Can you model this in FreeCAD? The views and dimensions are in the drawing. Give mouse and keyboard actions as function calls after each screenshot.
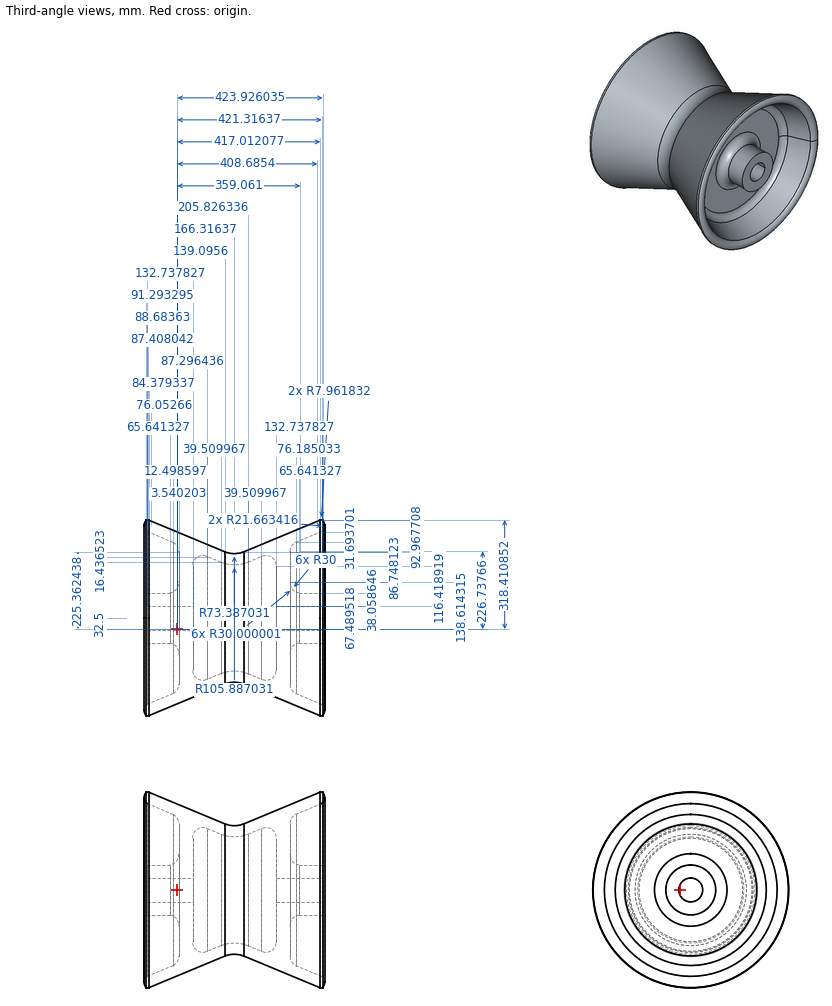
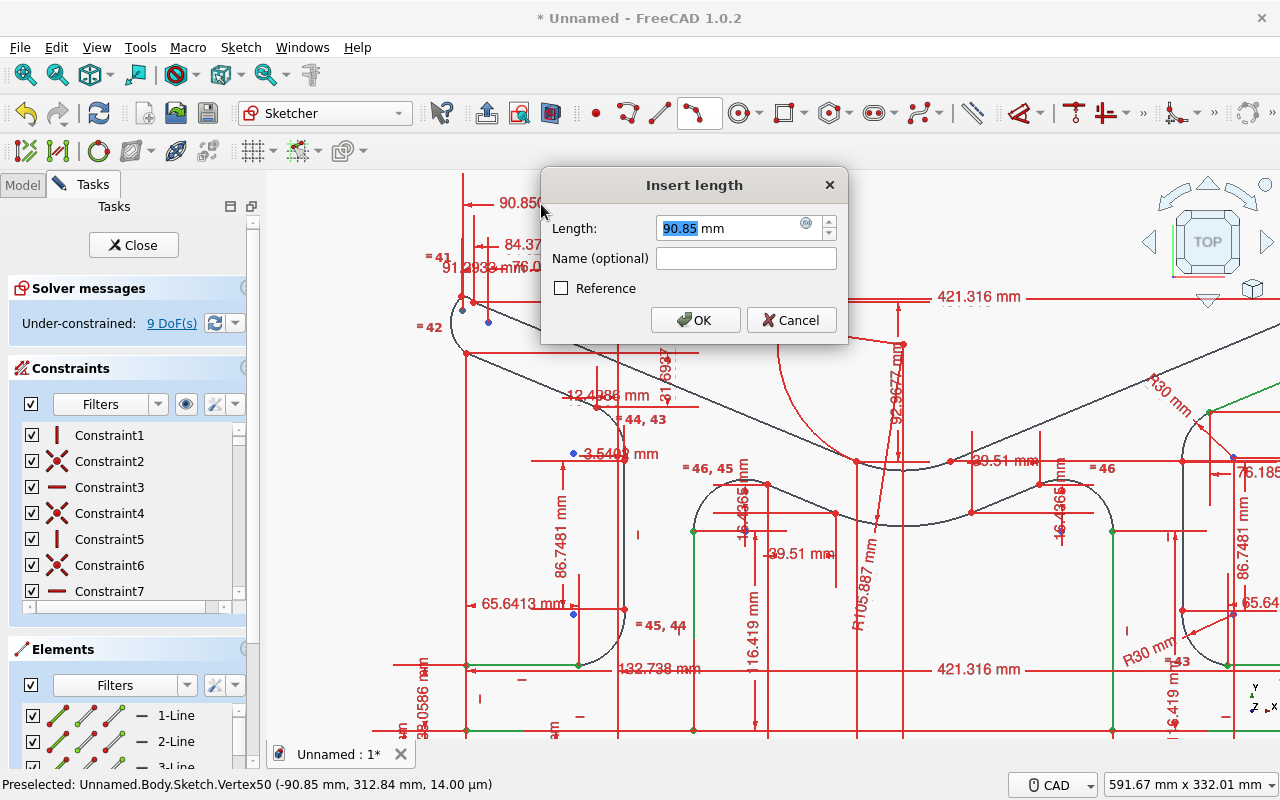
text(87.408042)
key(Return)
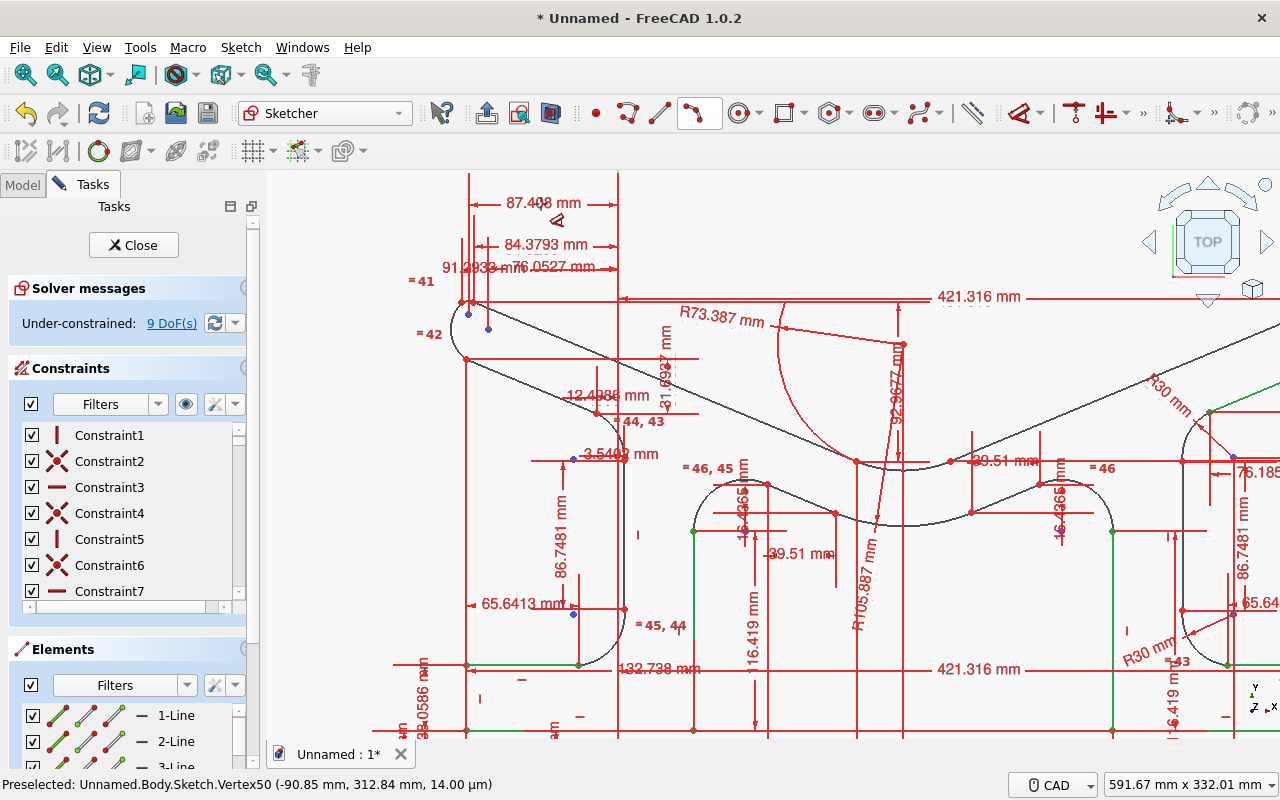
click(573, 459)
click(539, 643)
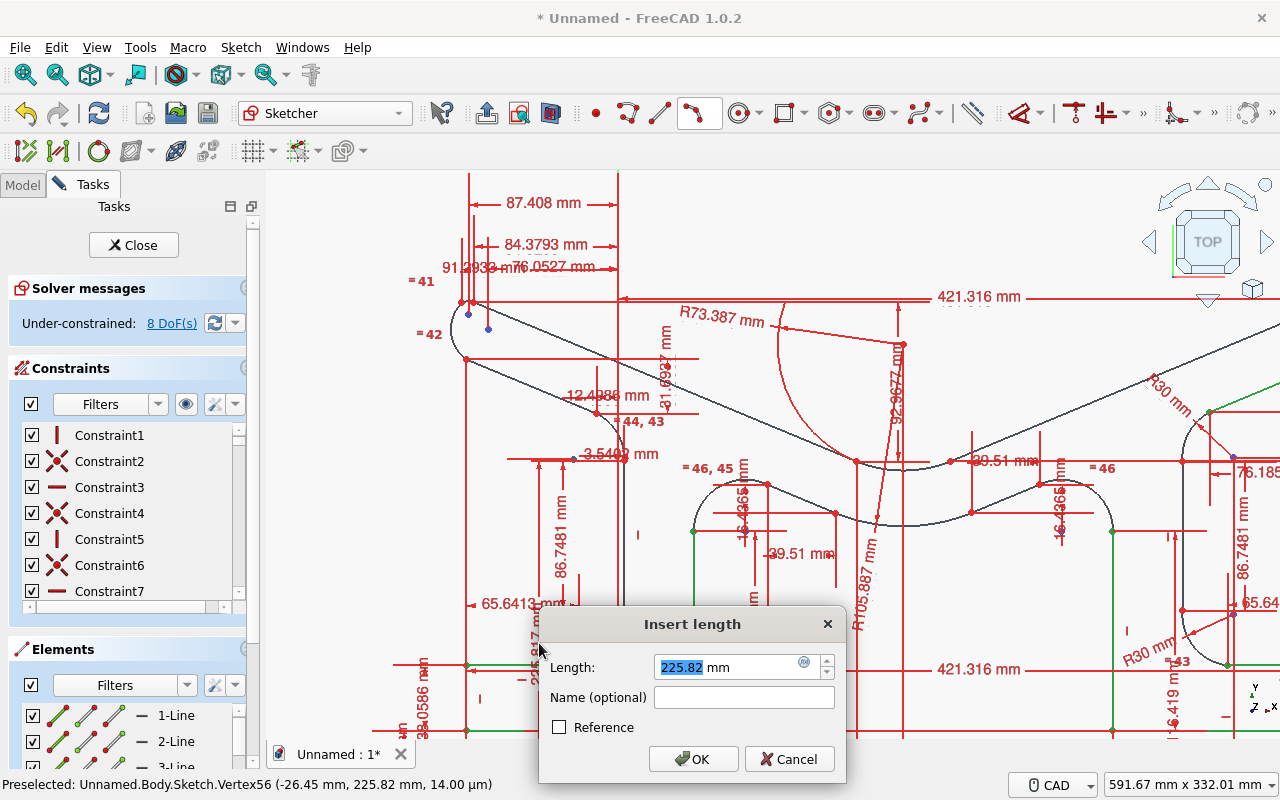
text(226.73766)
key(Return)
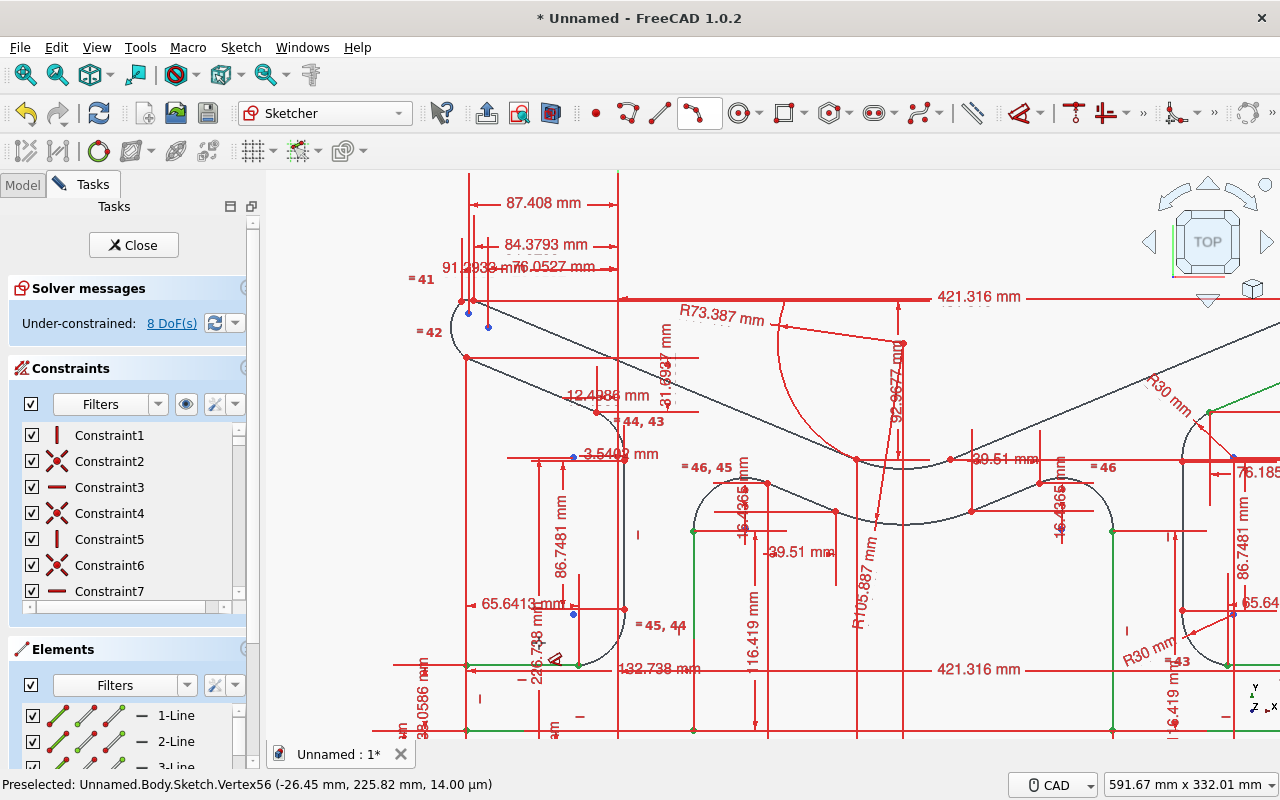
scroll(463, 310, down, 3)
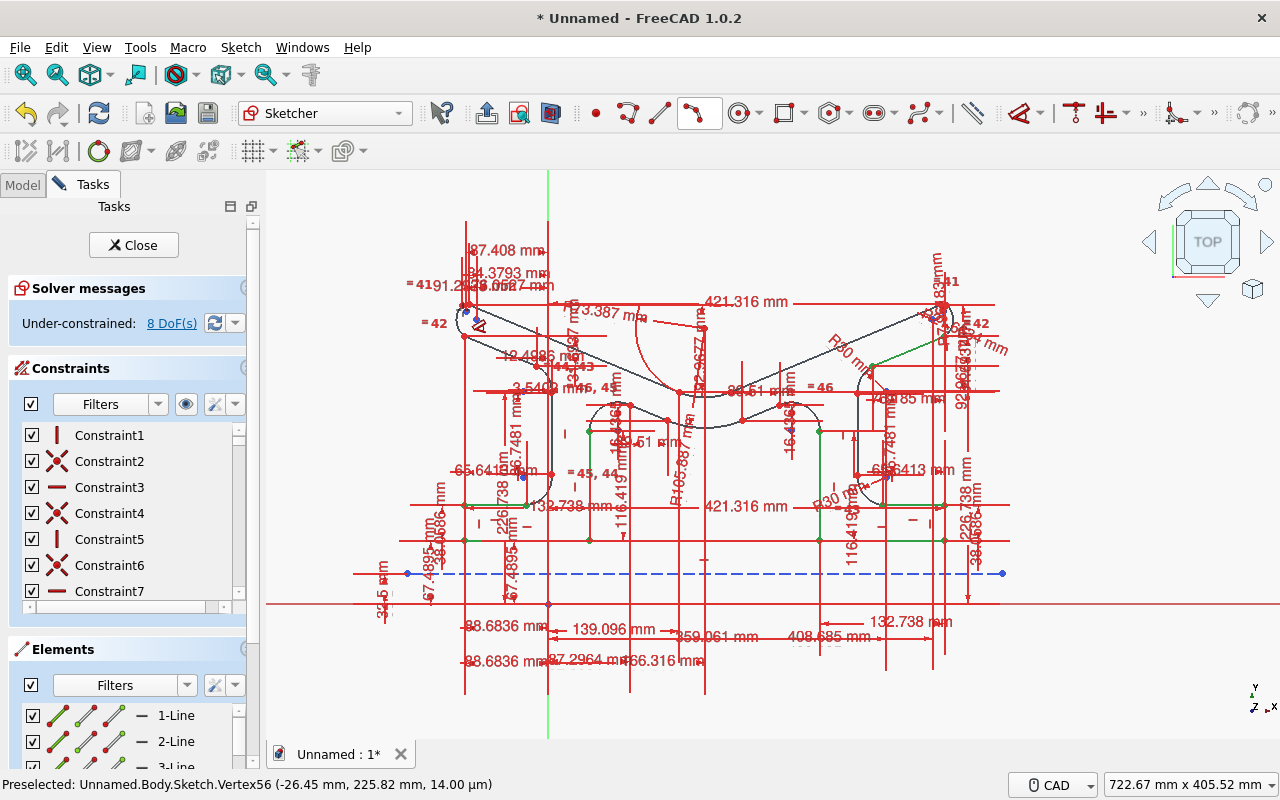
click(858, 475)
click(418, 495)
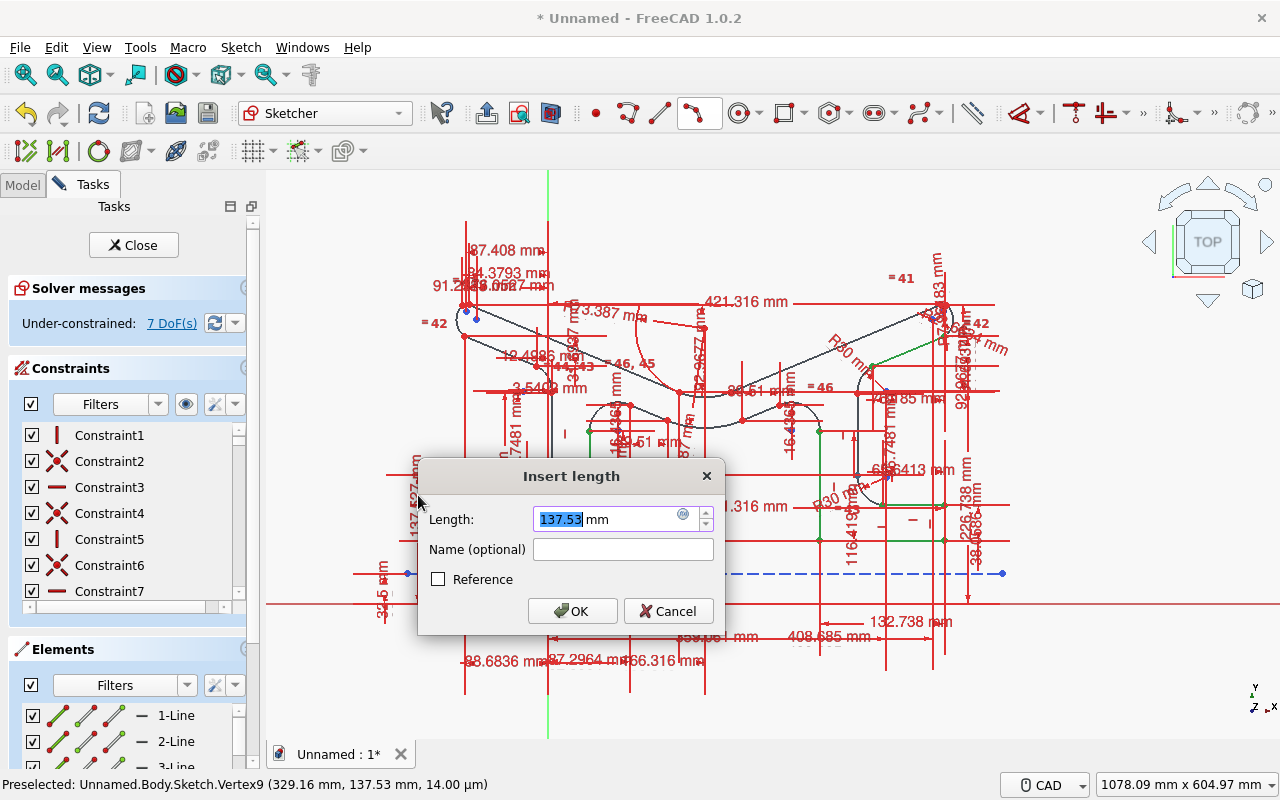
text(138.614315)
key(Return)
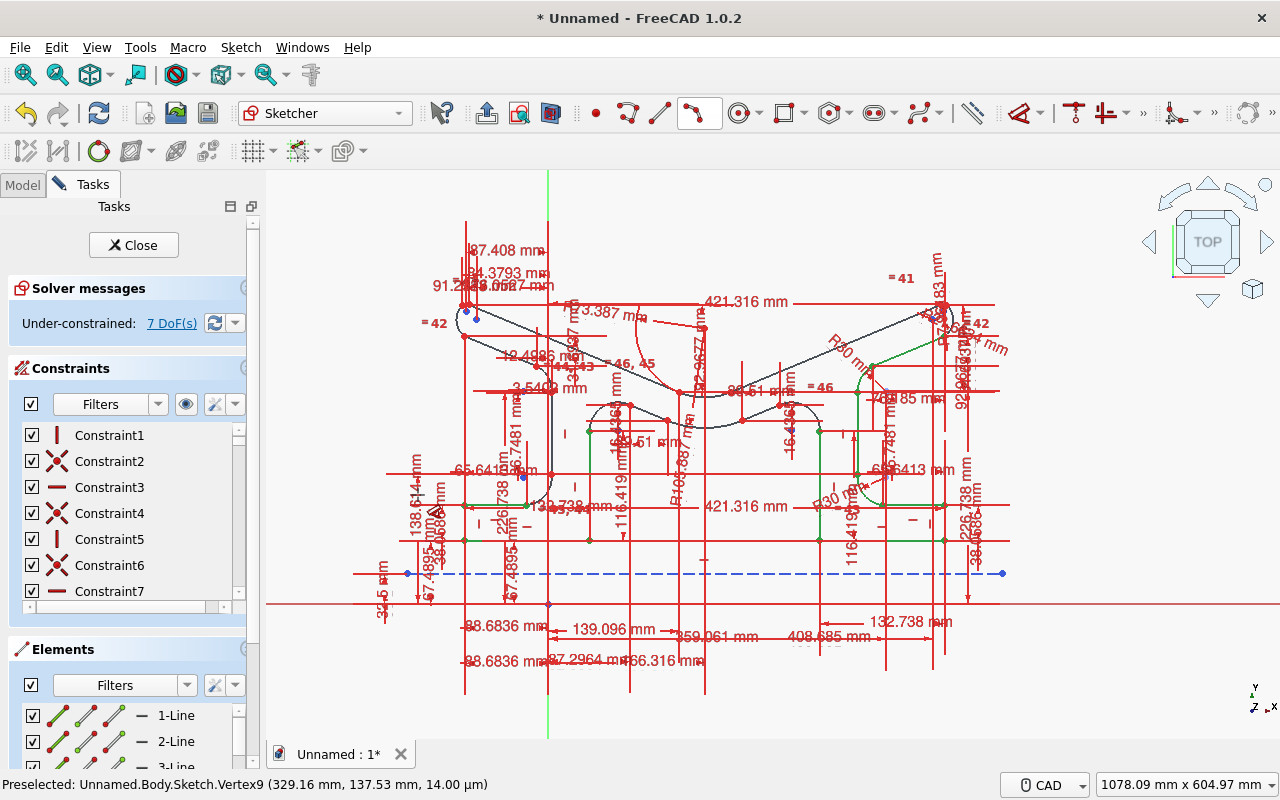
scroll(941, 305, up, 4)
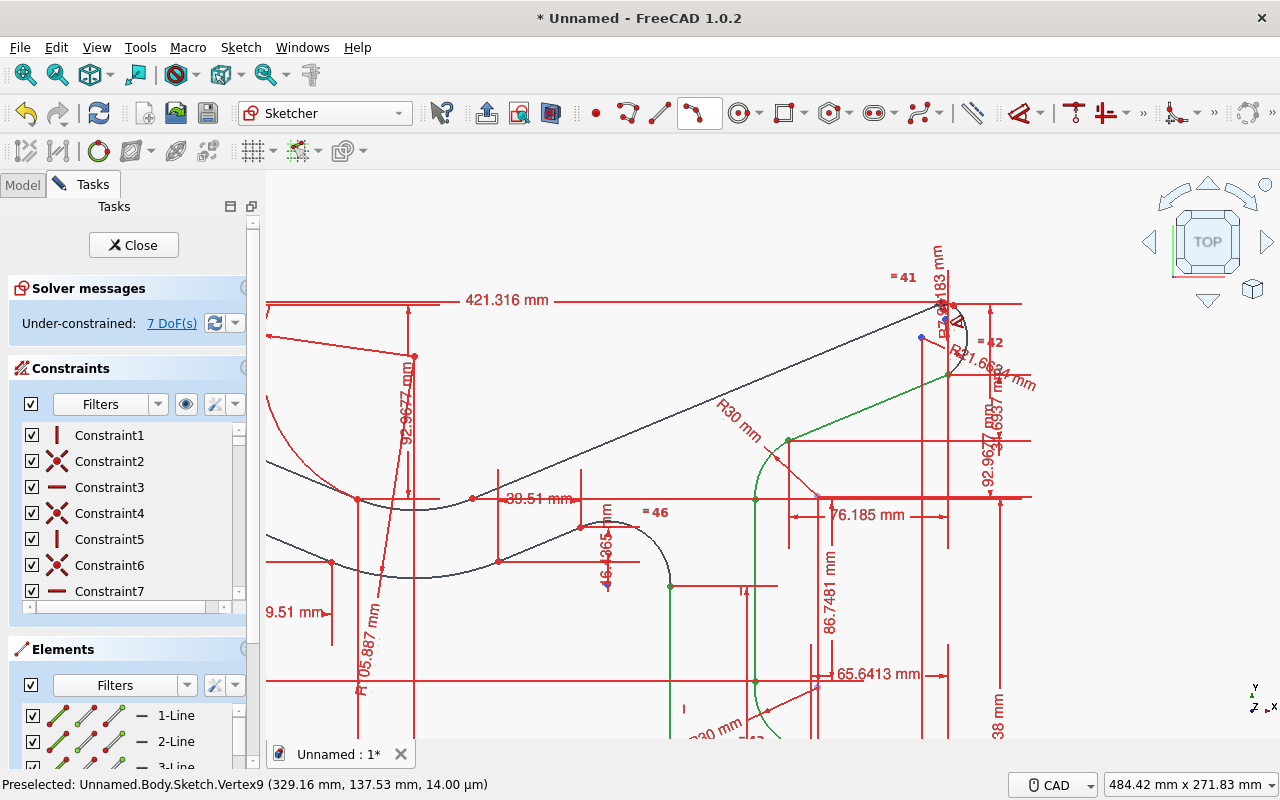
click(940, 304)
click(617, 270)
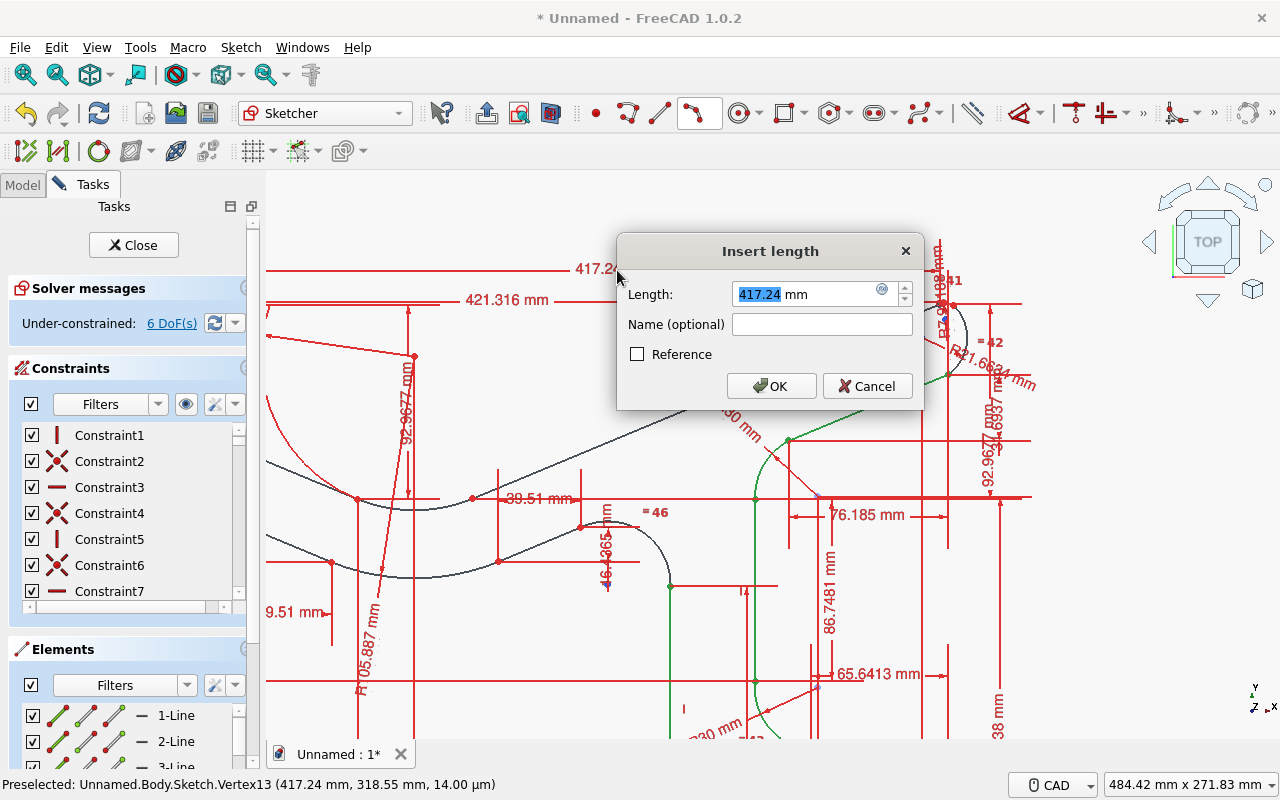
text(417.012077)
key(Return)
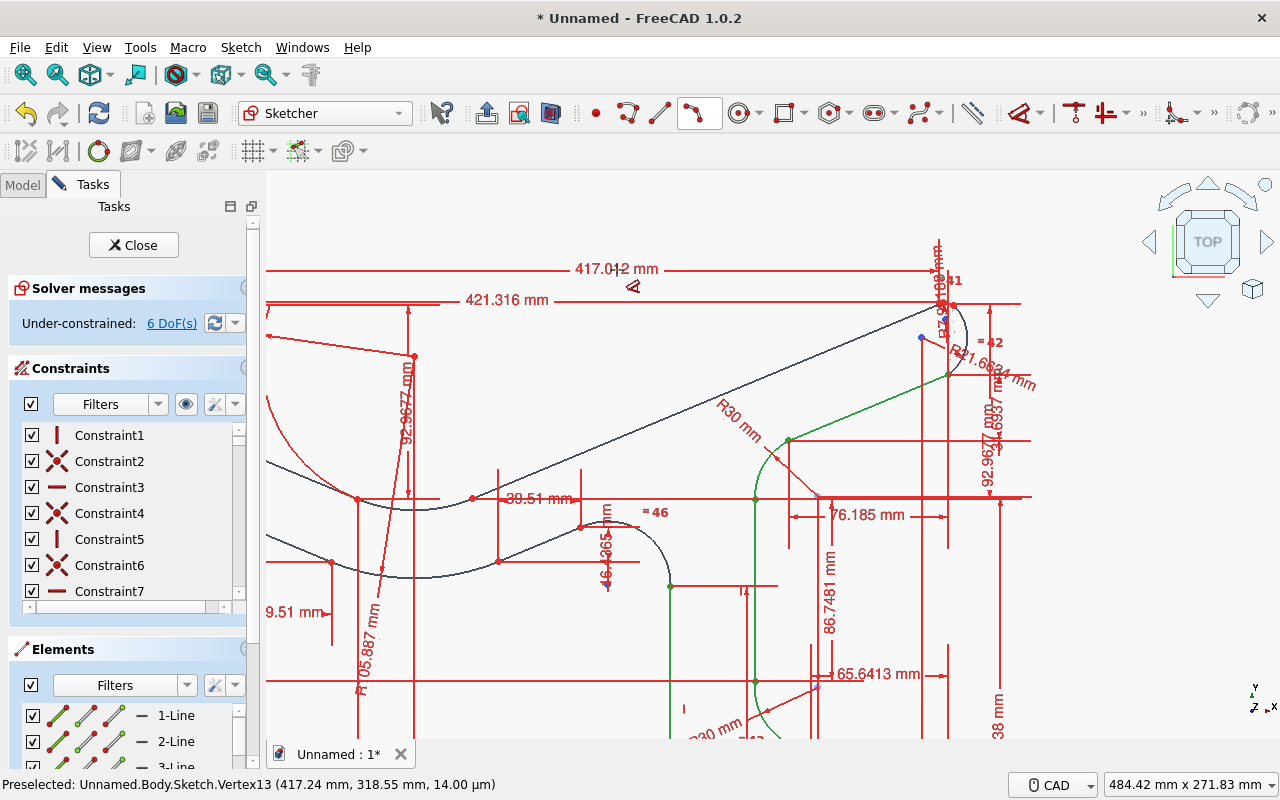
click(939, 304)
click(973, 508)